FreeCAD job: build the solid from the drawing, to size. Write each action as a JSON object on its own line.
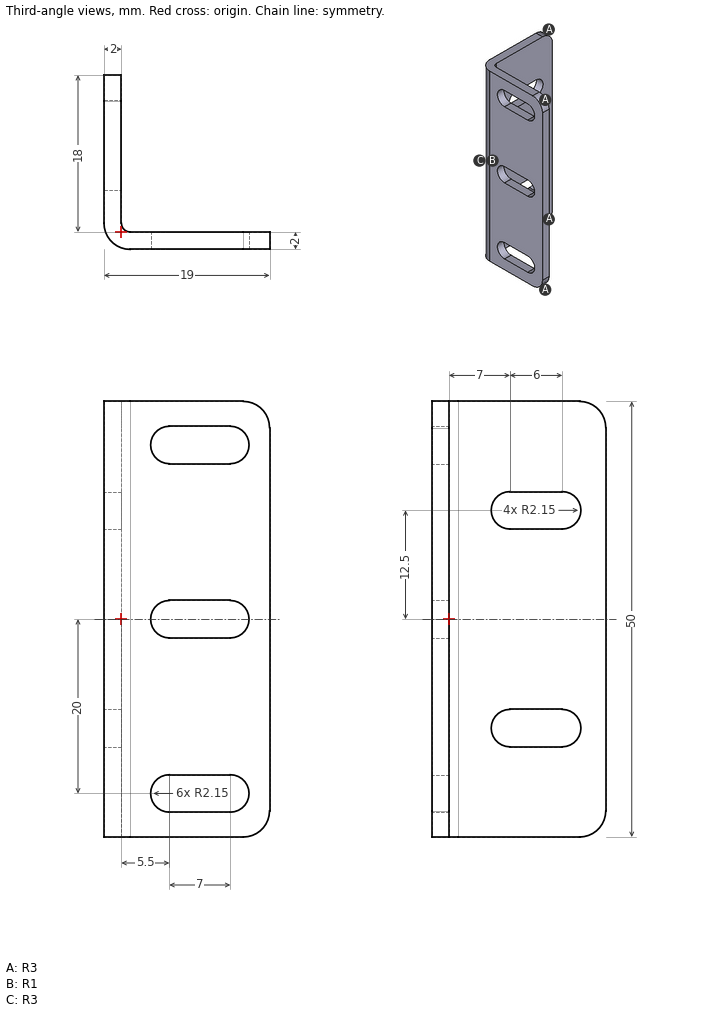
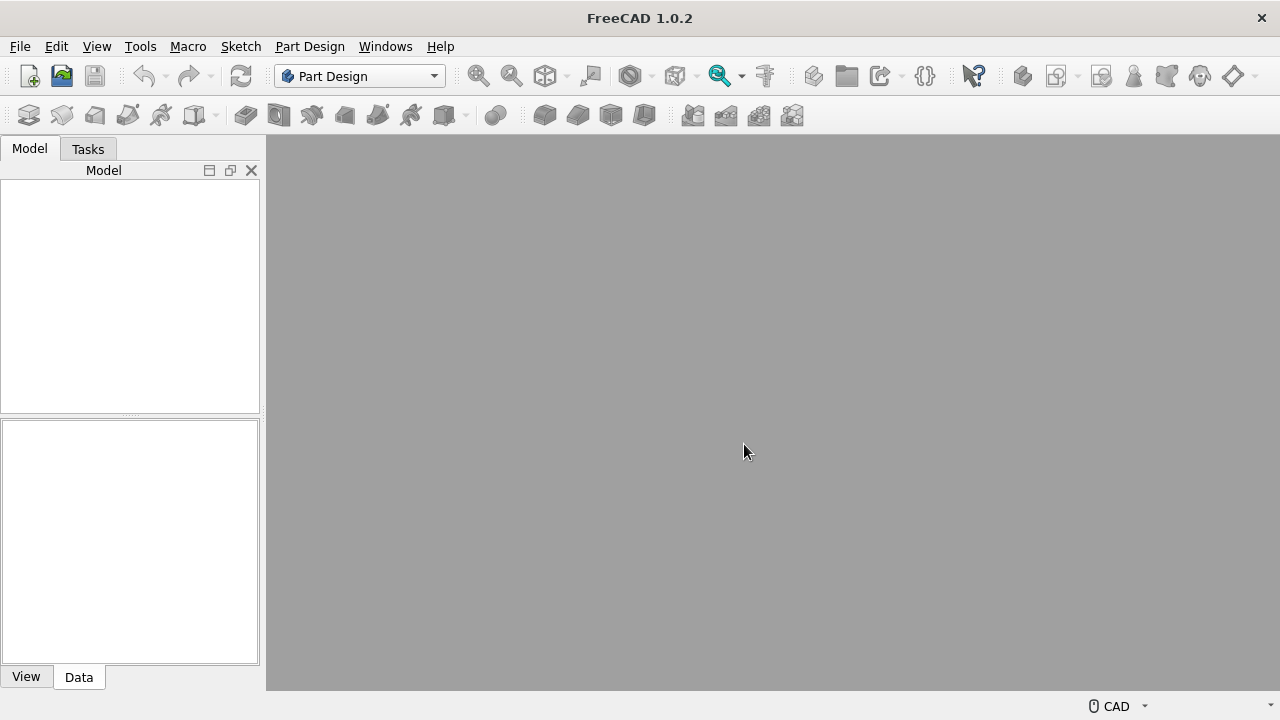
{"action": "left_click", "coordinate": [29, 76]}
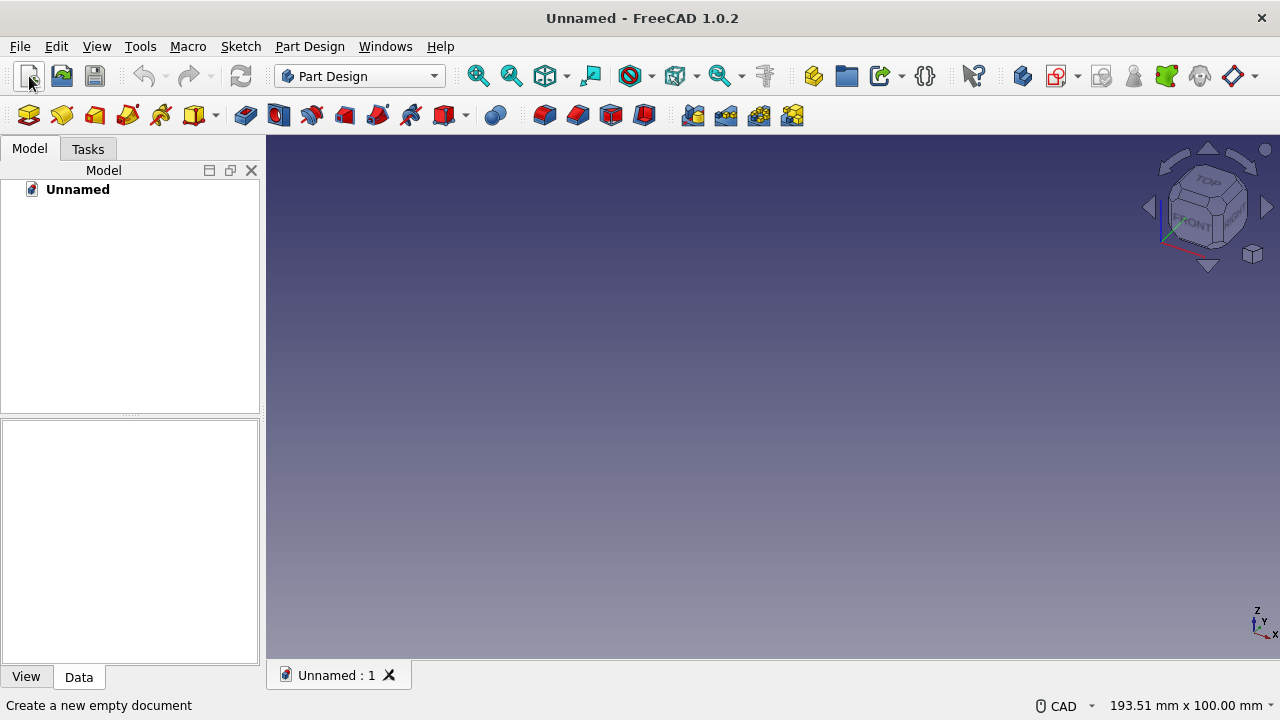
{"action": "left_click", "coordinate": [1056, 76]}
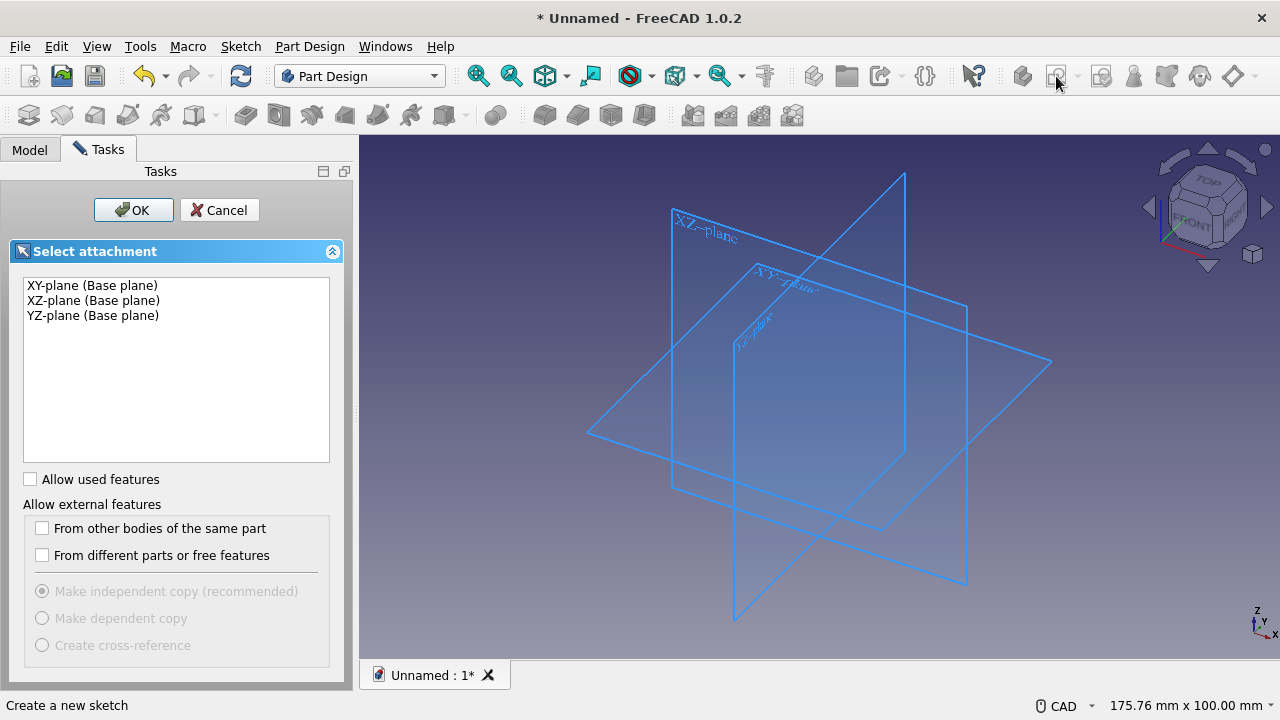
{"action": "left_click", "coordinate": [84, 286]}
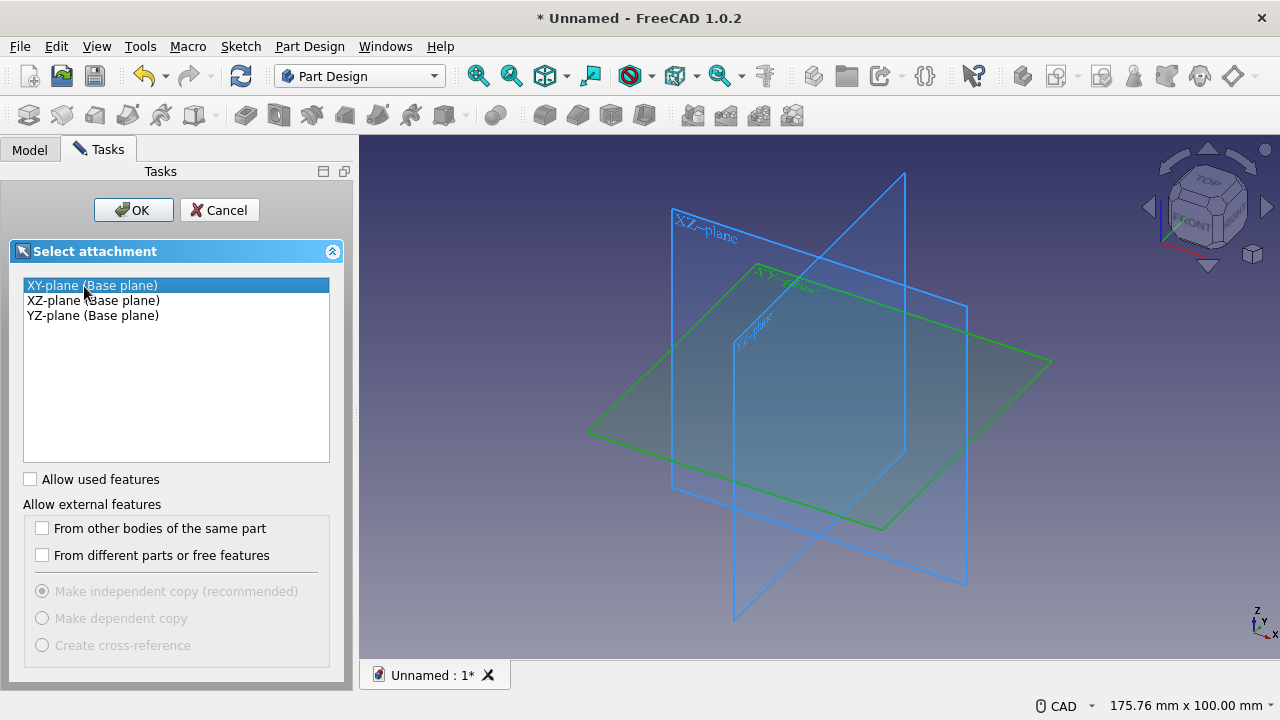
{"action": "left_click", "coordinate": [134, 210]}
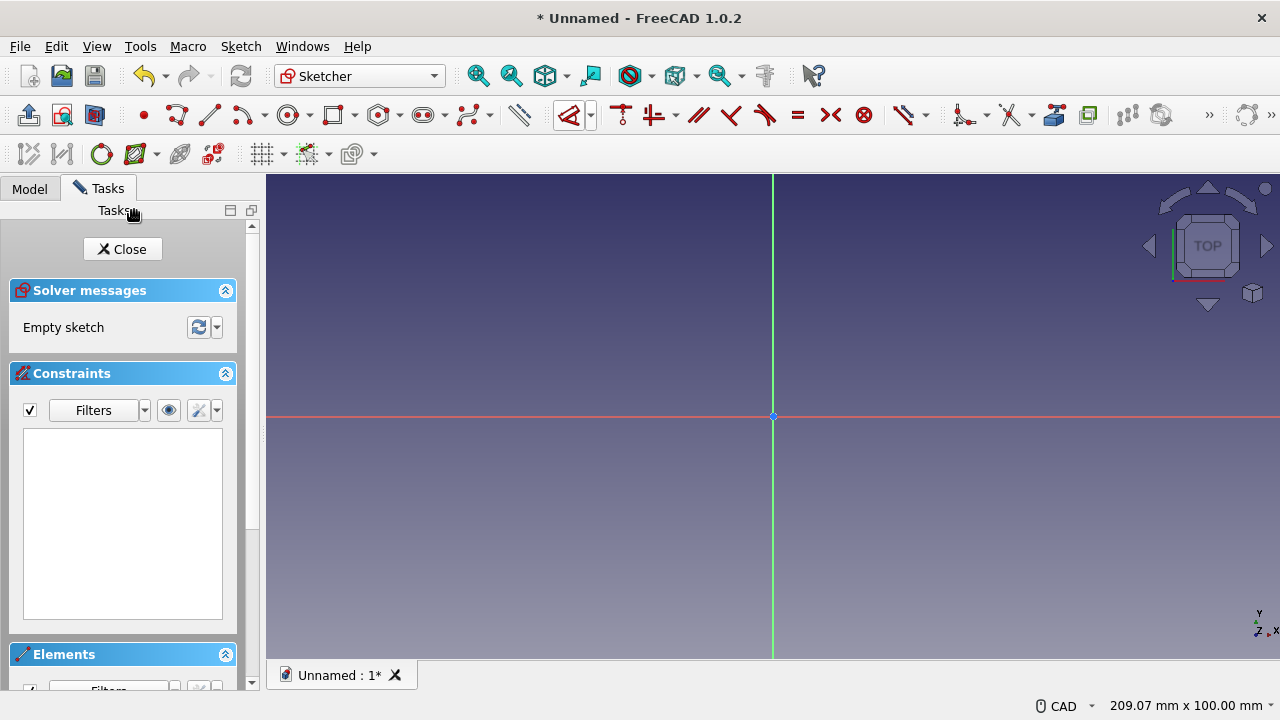
{"action": "scroll", "coordinate": [855, 361], "scroll_direction": "up", "scroll_amount": 6}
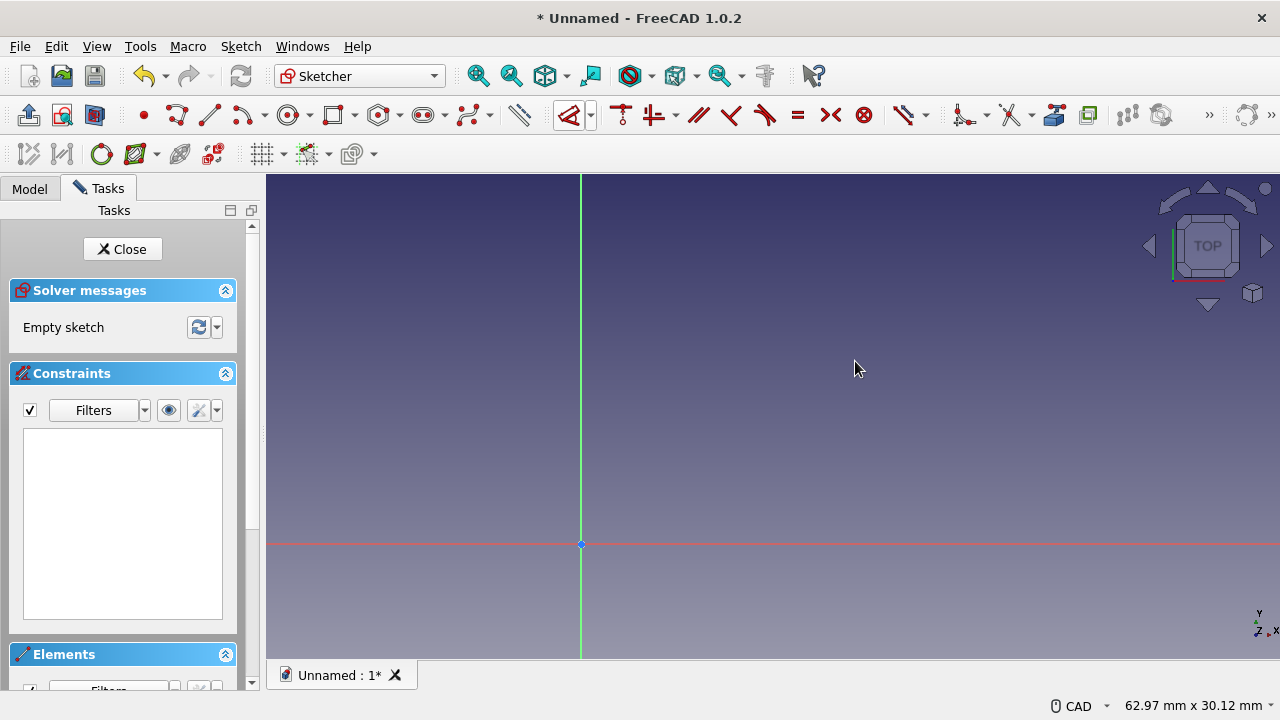
{"action": "left_click", "coordinate": [177, 116]}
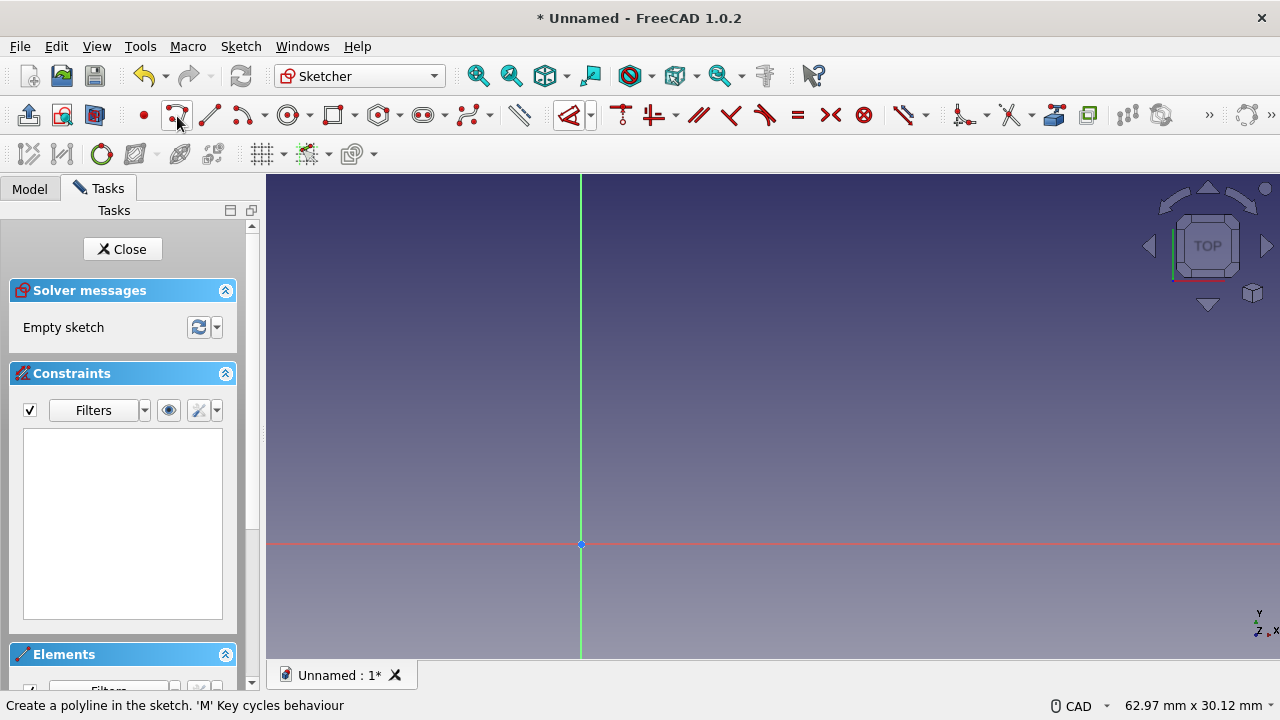
{"action": "left_click", "coordinate": [581, 544]}
{"action": "left_click", "coordinate": [590, 255]}
{"action": "left_click", "coordinate": [549, 255]}
{"action": "left_click", "coordinate": [549, 577]}
{"action": "left_click", "coordinate": [855, 577]}
{"action": "left_click", "coordinate": [855, 535]}
{"action": "left_click", "coordinate": [581, 544]}
{"action": "key", "text": "Escape"}
{"action": "key", "text": "Escape"}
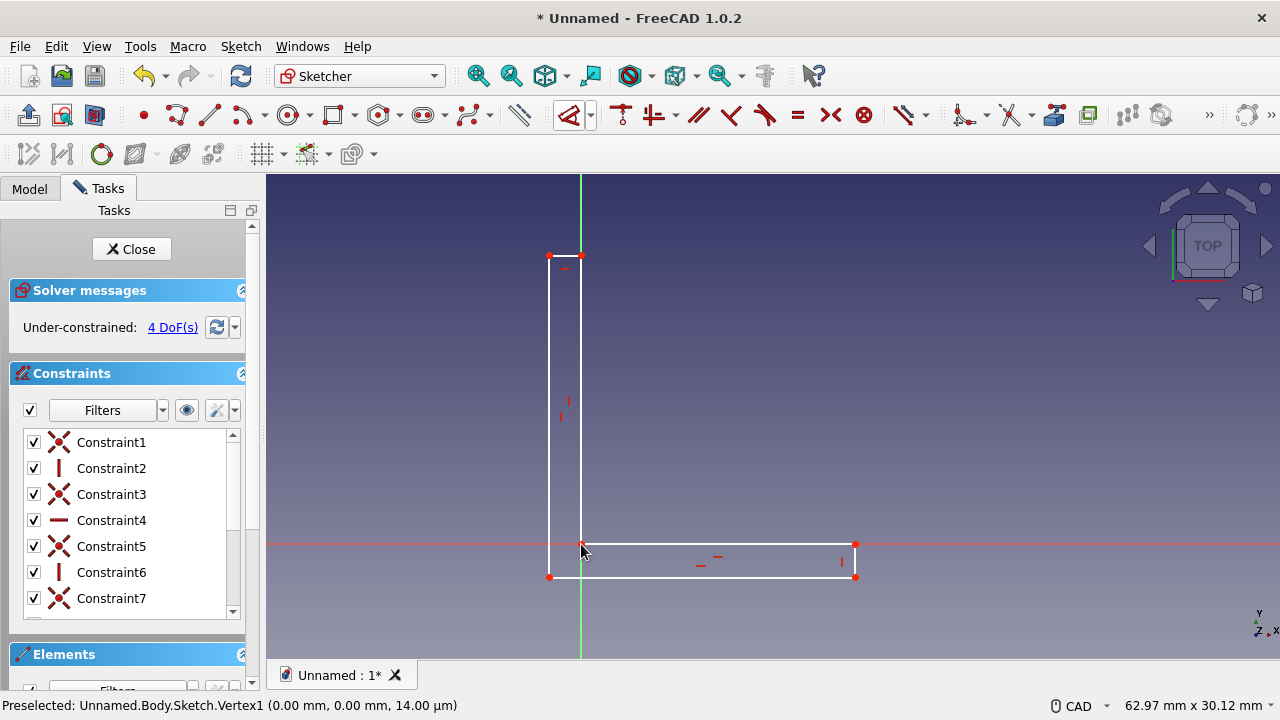
{"action": "left_click", "coordinate": [568, 116]}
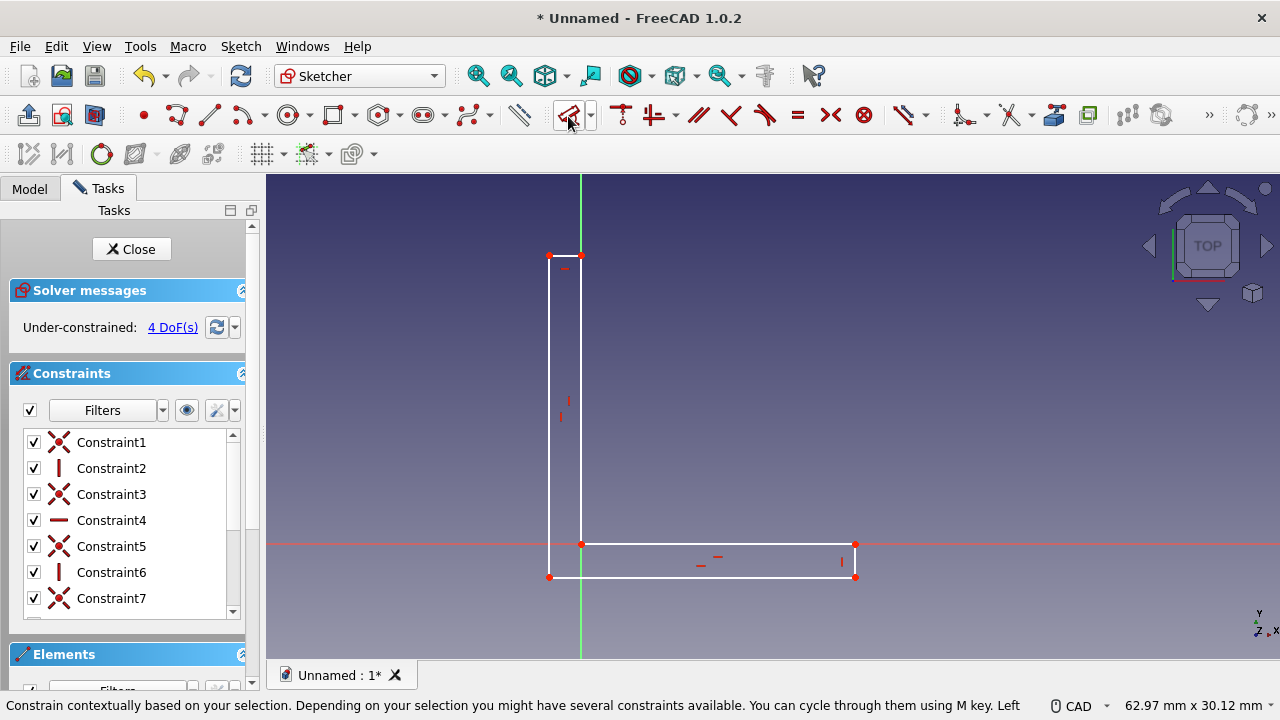
{"action": "scroll", "coordinate": [572, 256], "scroll_direction": "up", "scroll_amount": 2}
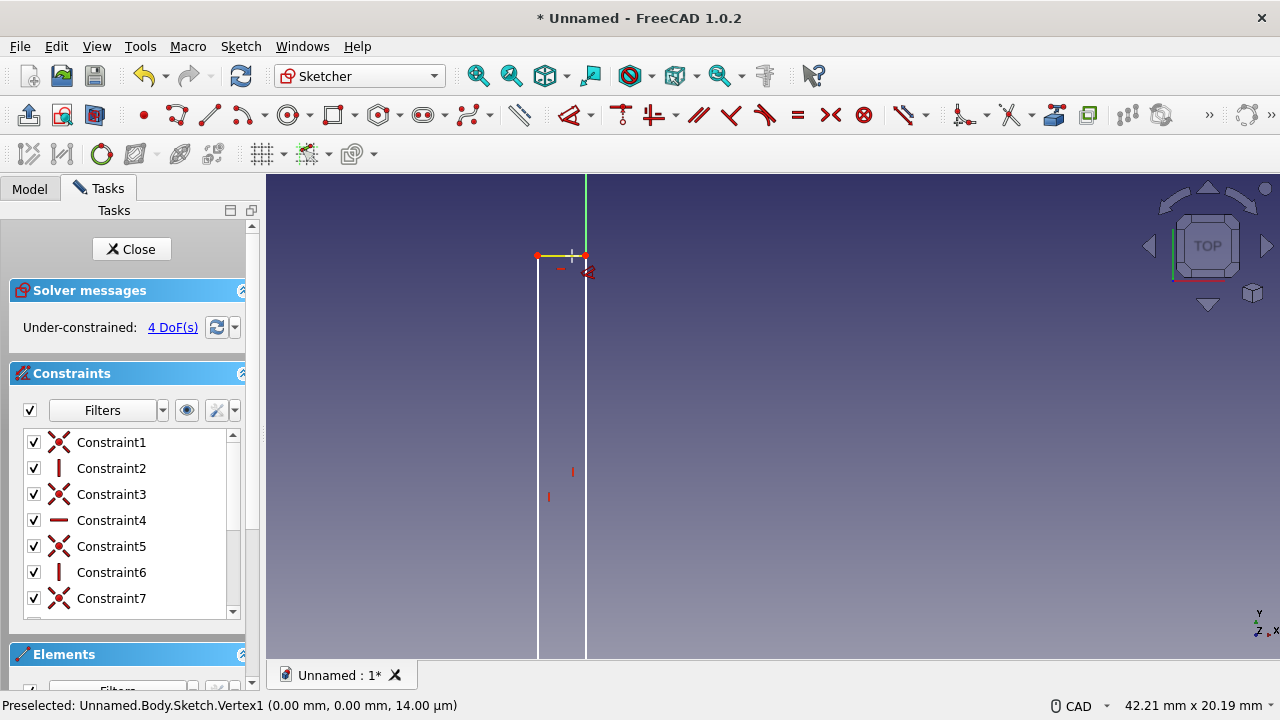
{"action": "left_click", "coordinate": [571, 256]}
{"action": "left_click", "coordinate": [562, 222]}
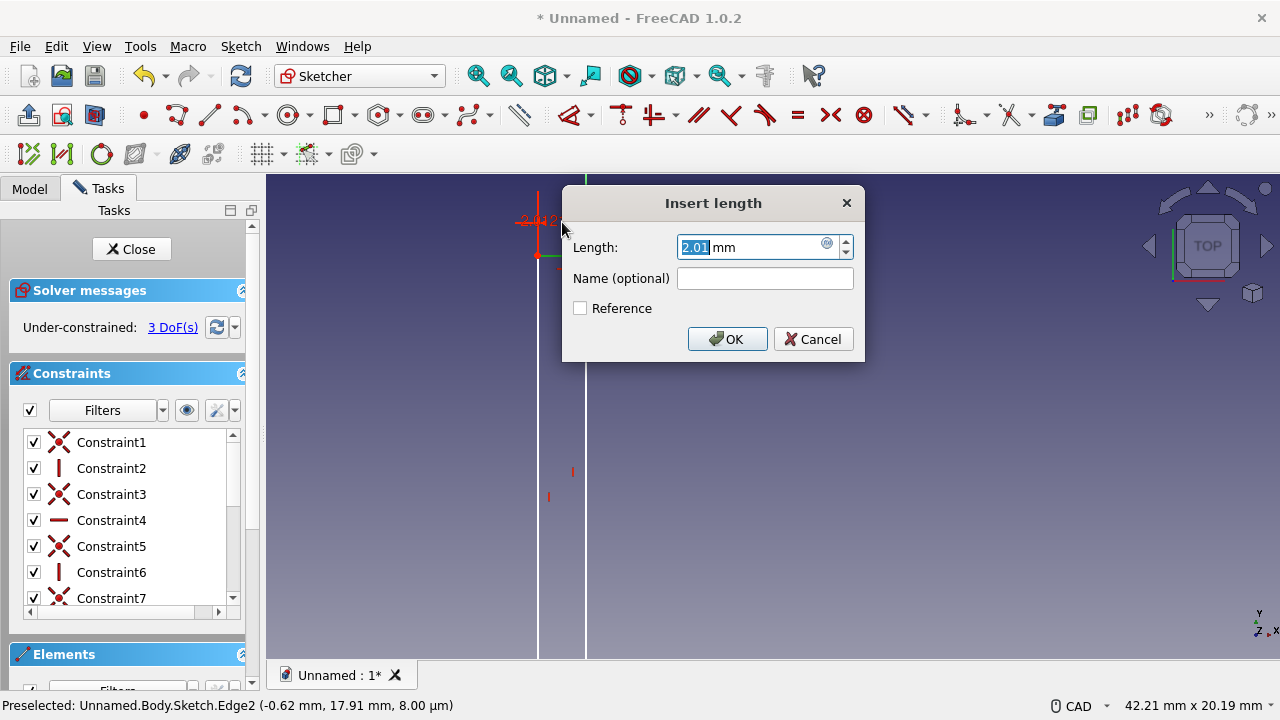
{"action": "type", "text": "2"}
{"action": "key", "text": "Return"}